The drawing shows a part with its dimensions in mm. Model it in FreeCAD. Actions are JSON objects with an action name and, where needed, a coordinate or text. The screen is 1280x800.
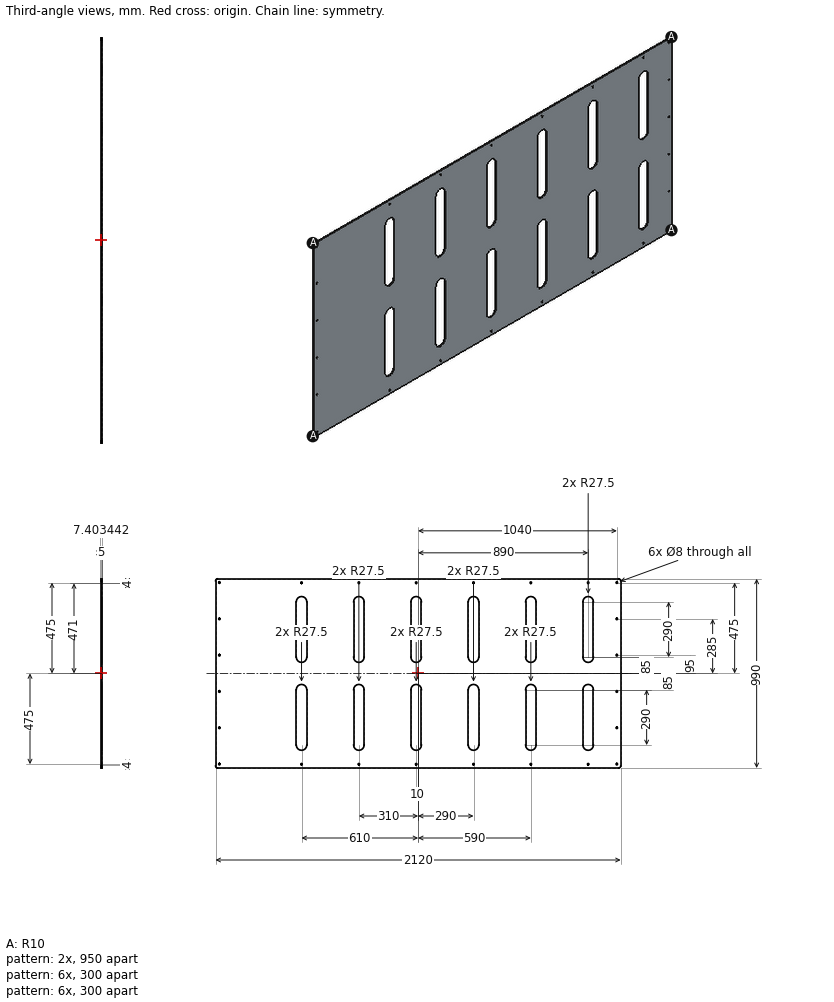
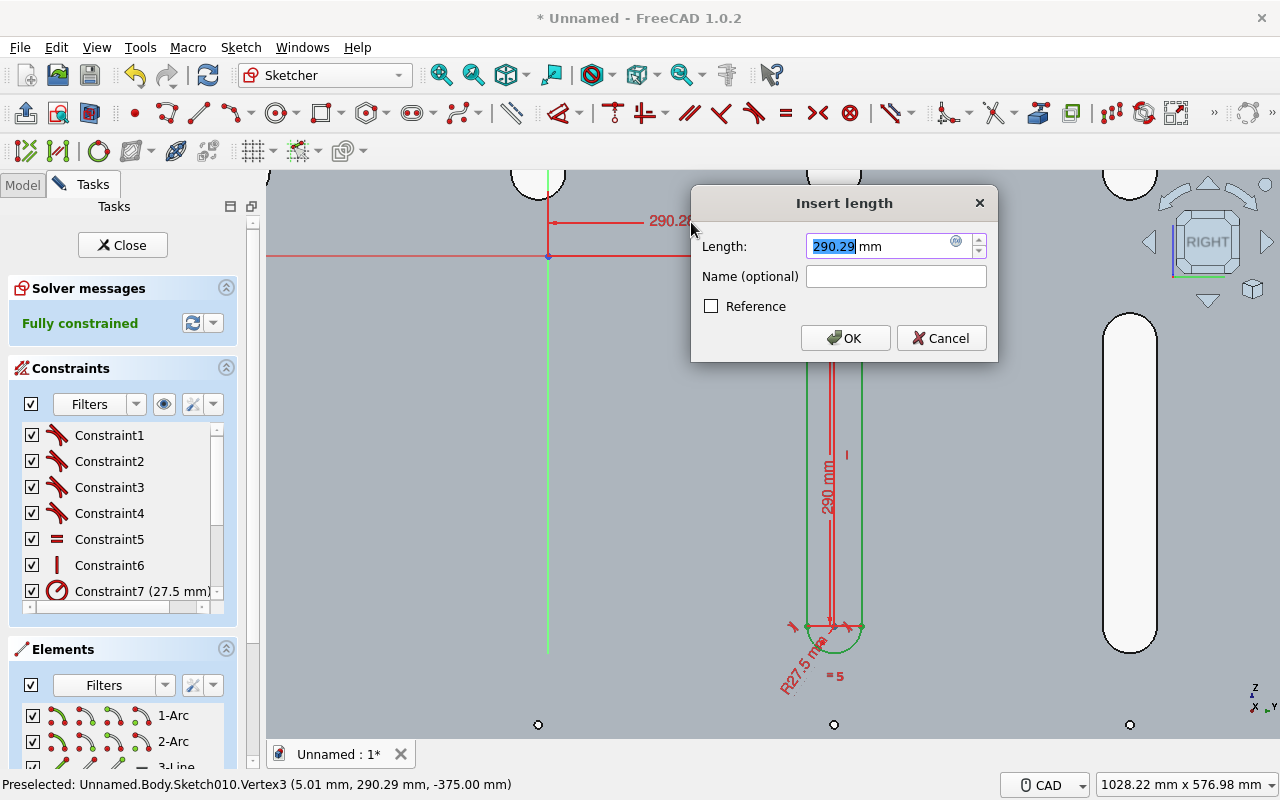
{"action": "type", "text": "290"}
{"action": "key", "text": "Return"}
{"action": "key", "text": "Escape"}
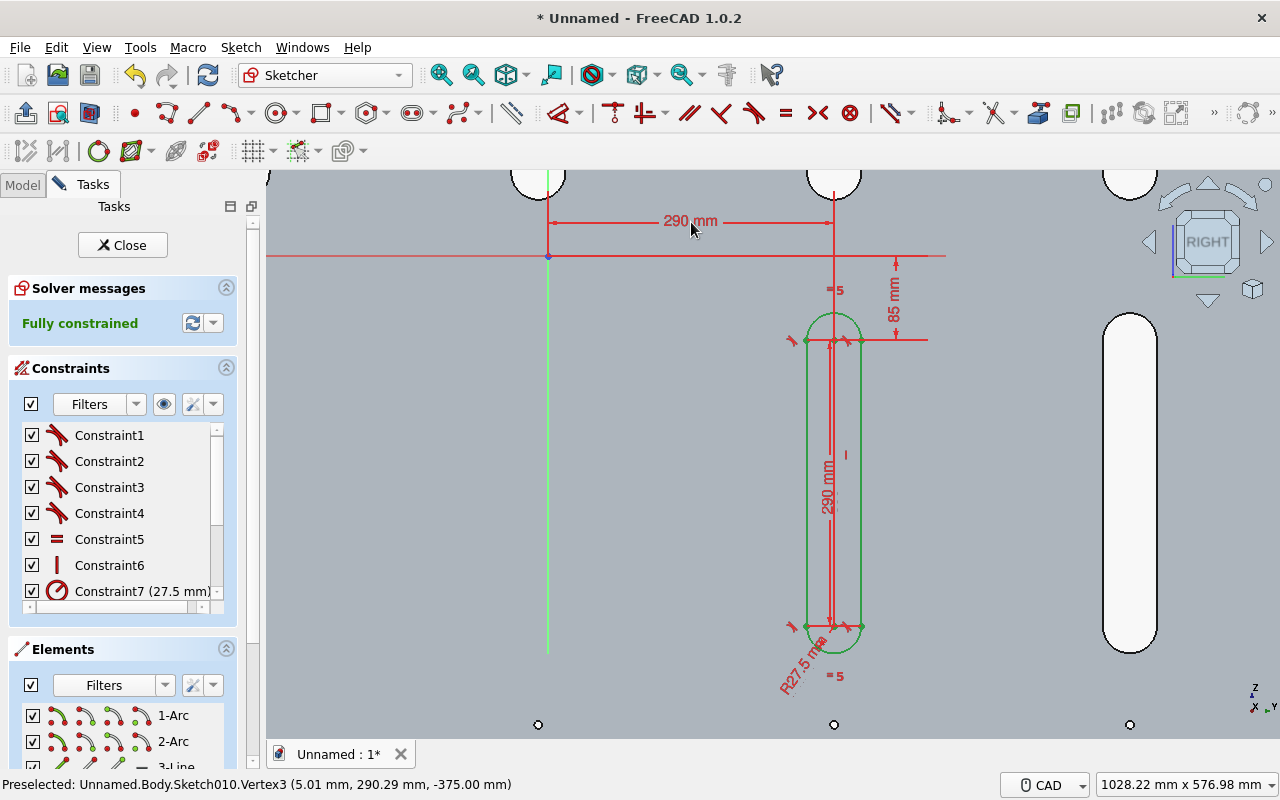
{"action": "left_click", "coordinate": [123, 245]}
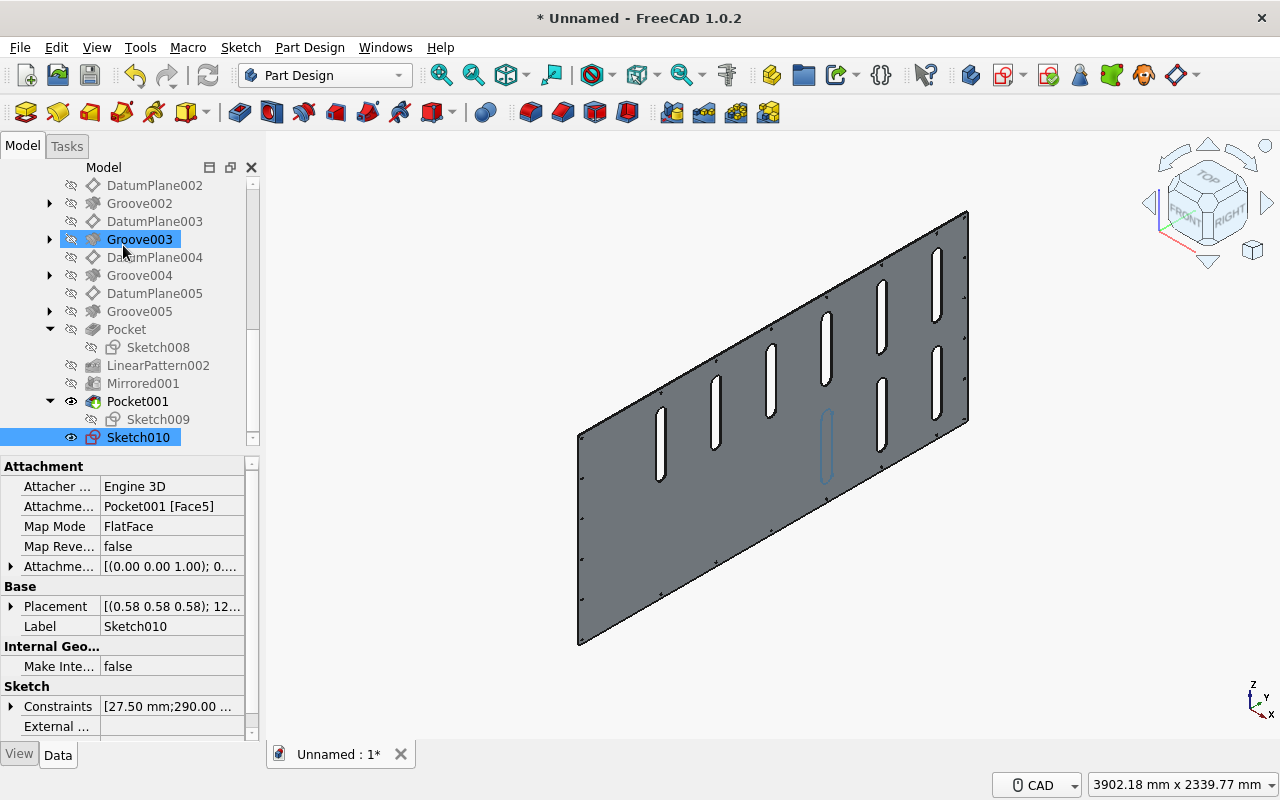
{"action": "left_click", "coordinate": [240, 112]}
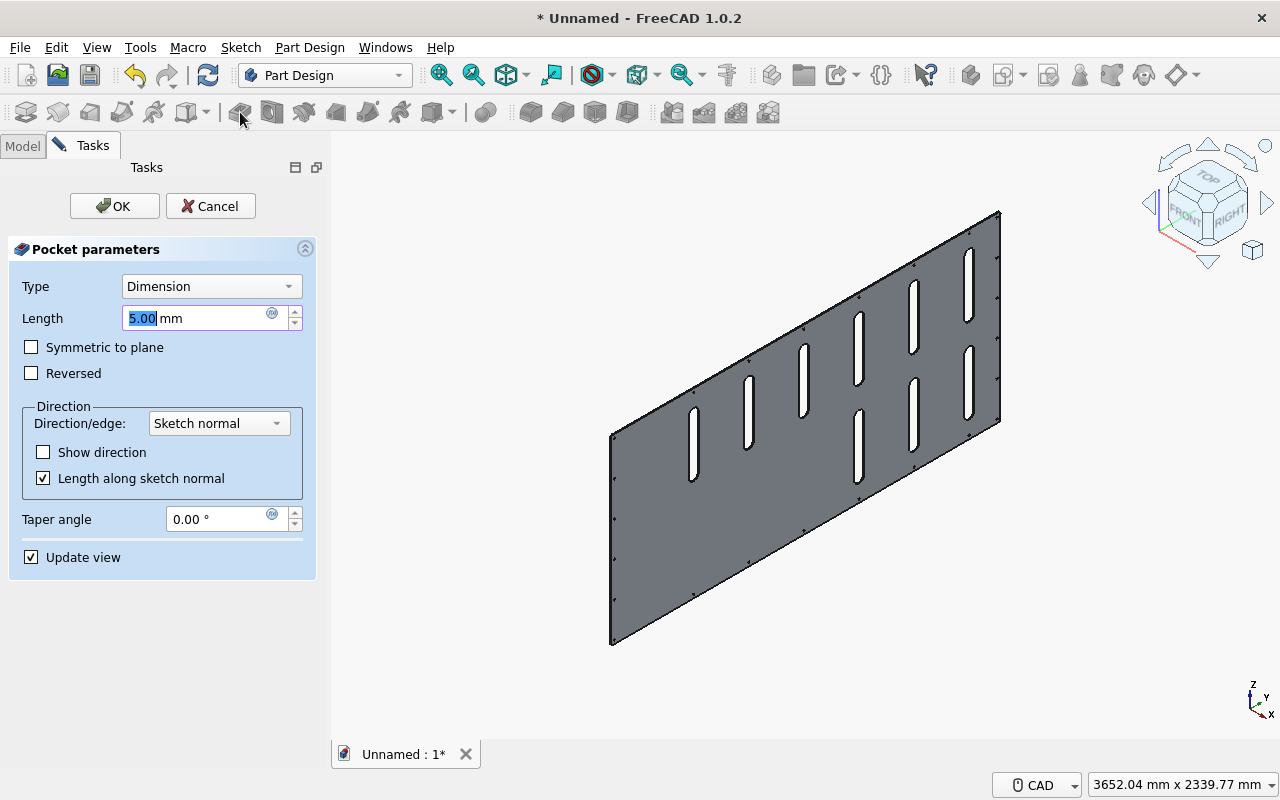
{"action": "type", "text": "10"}
{"action": "key", "text": "Tab"}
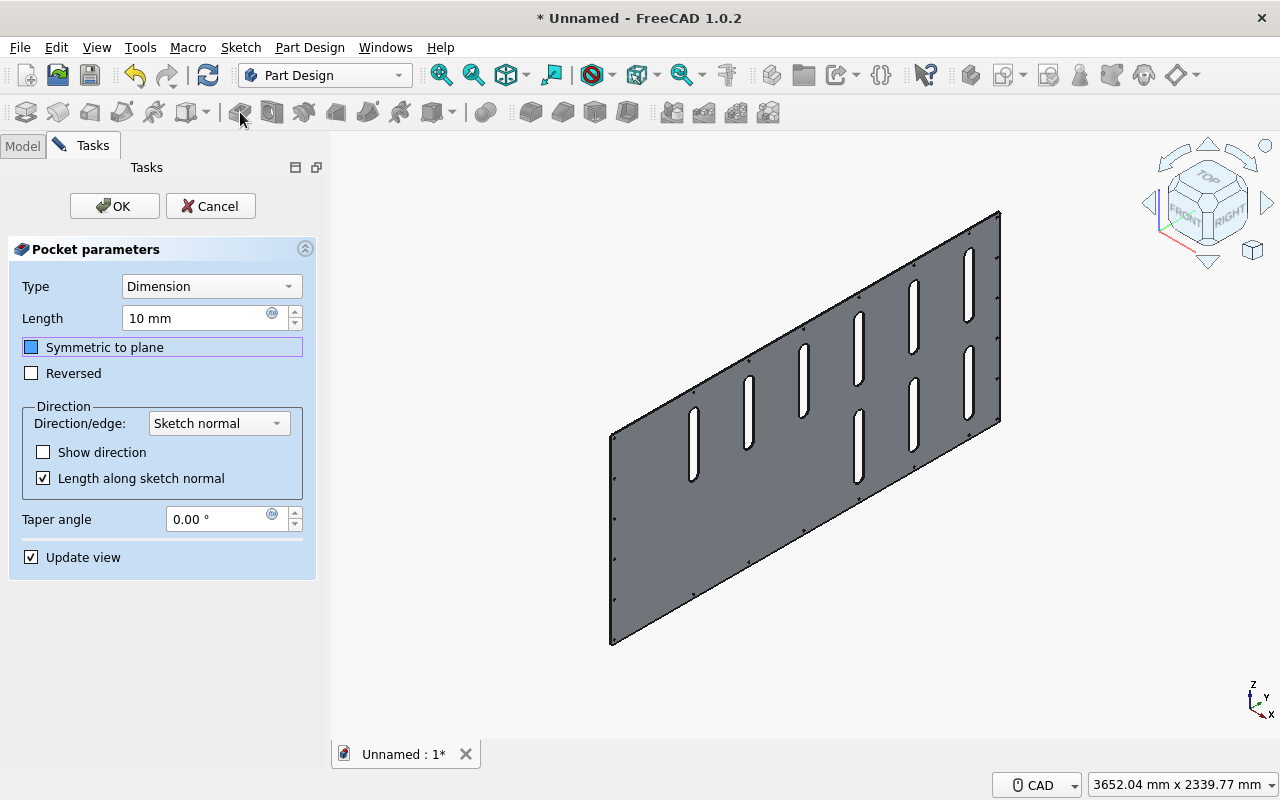
{"action": "left_click", "coordinate": [115, 206]}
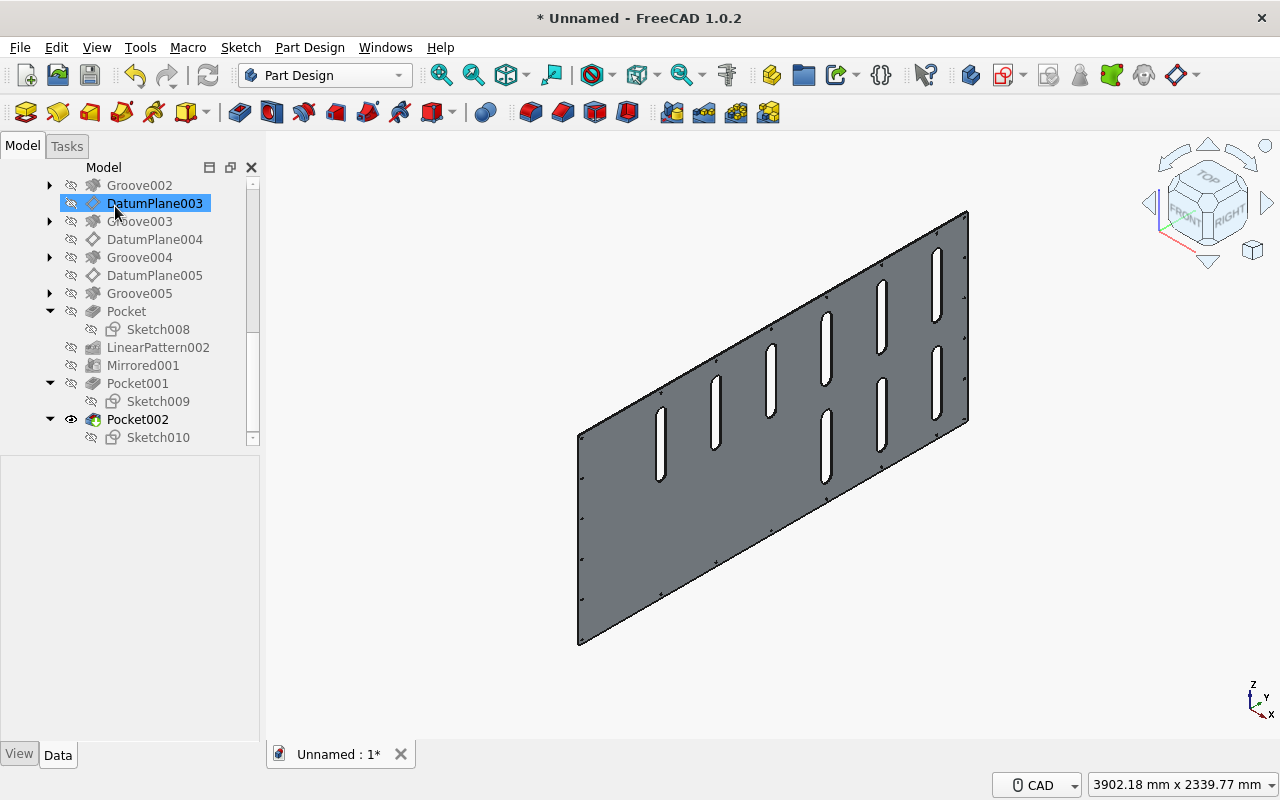
{"action": "left_click", "coordinate": [773, 458]}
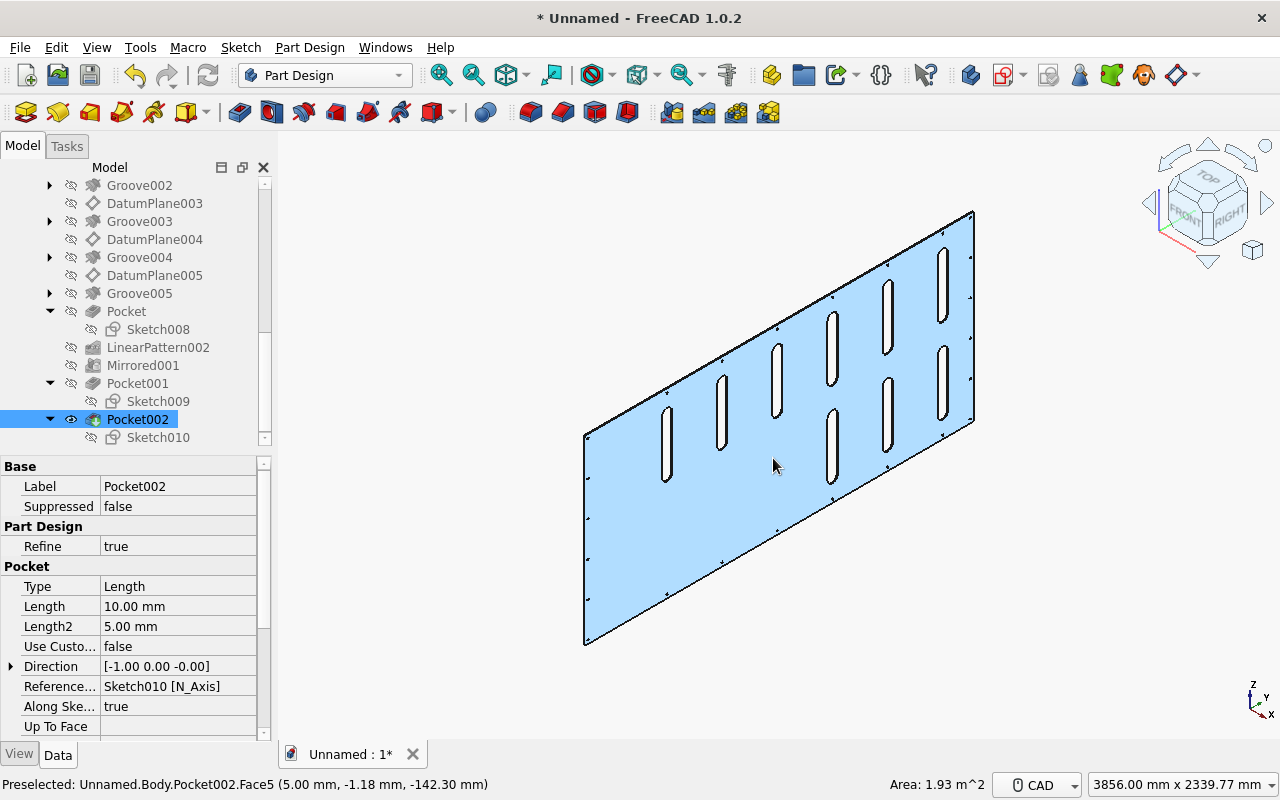
{"action": "left_click", "coordinate": [1004, 76]}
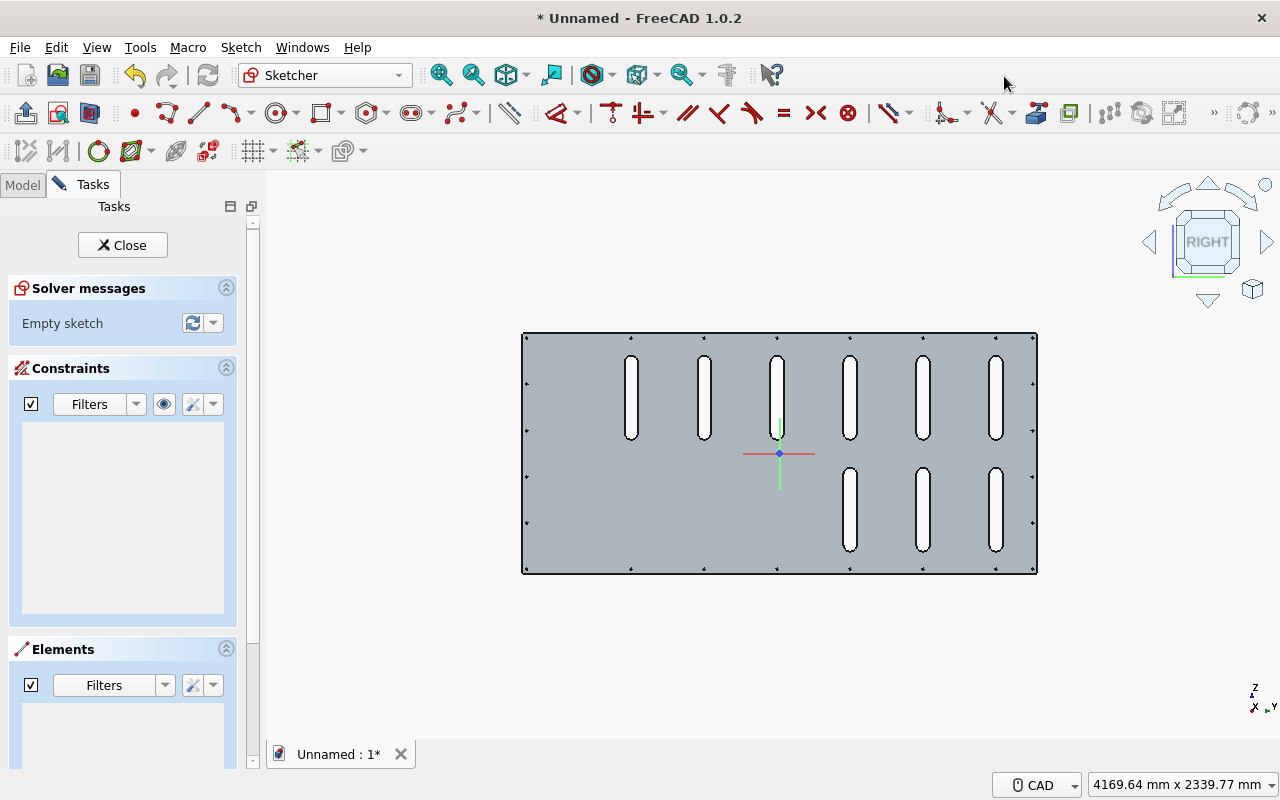
{"action": "scroll", "coordinate": [801, 518], "scroll_direction": "up", "scroll_amount": 7}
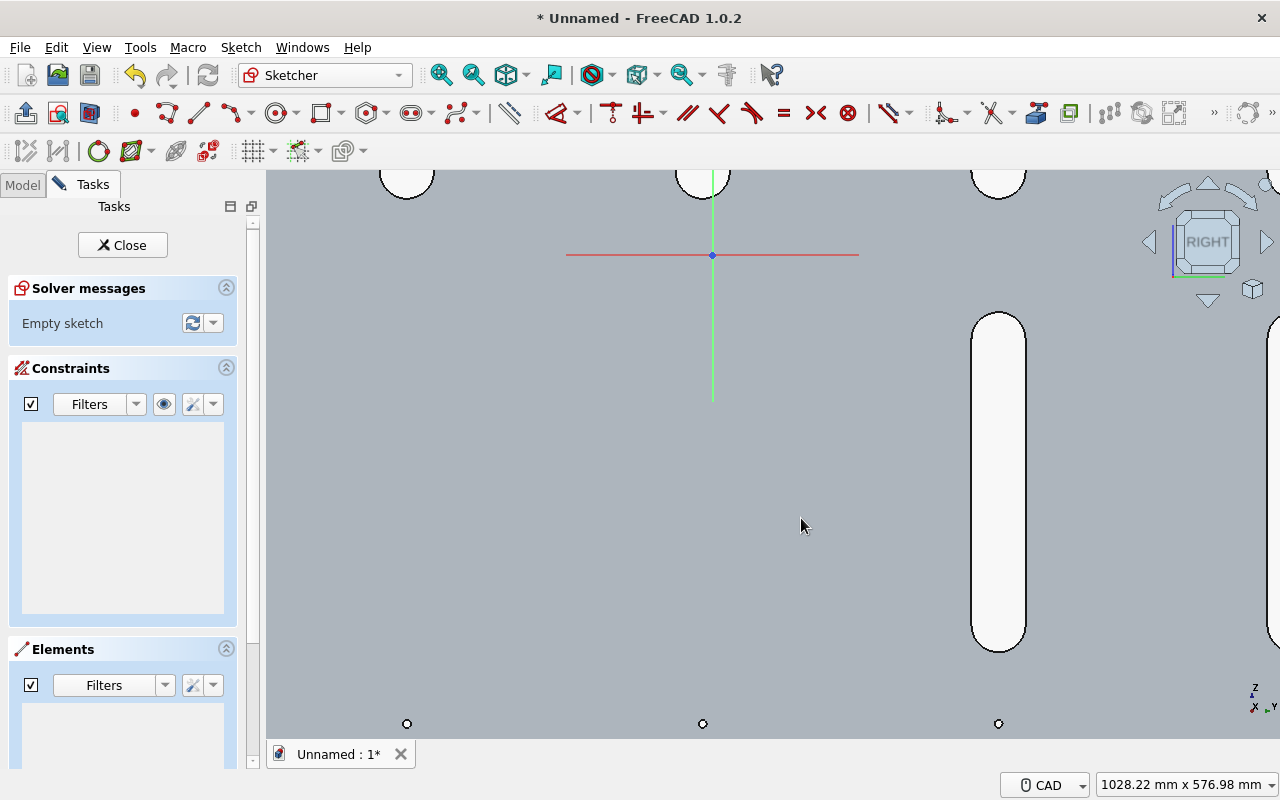
{"action": "left_click", "coordinate": [412, 114]}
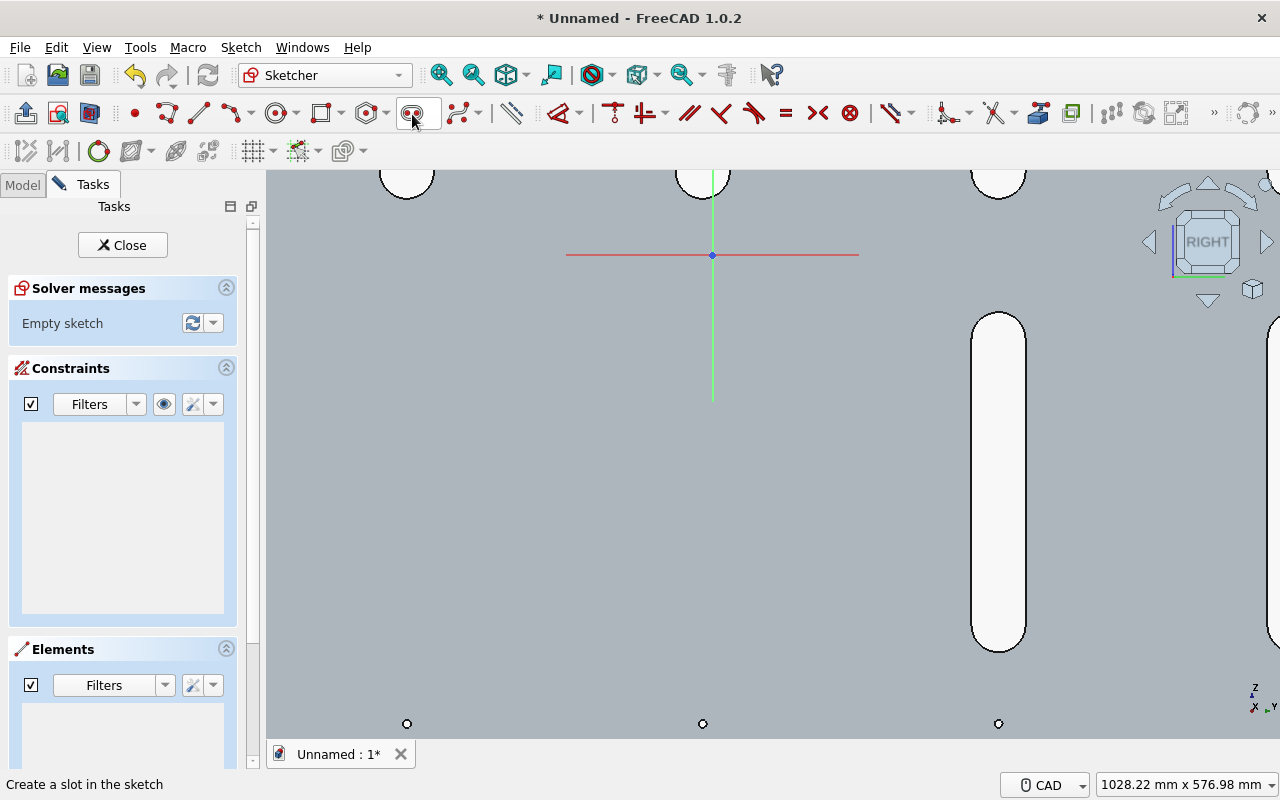
{"action": "scroll", "coordinate": [703, 625], "scroll_direction": "up", "scroll_amount": 3}